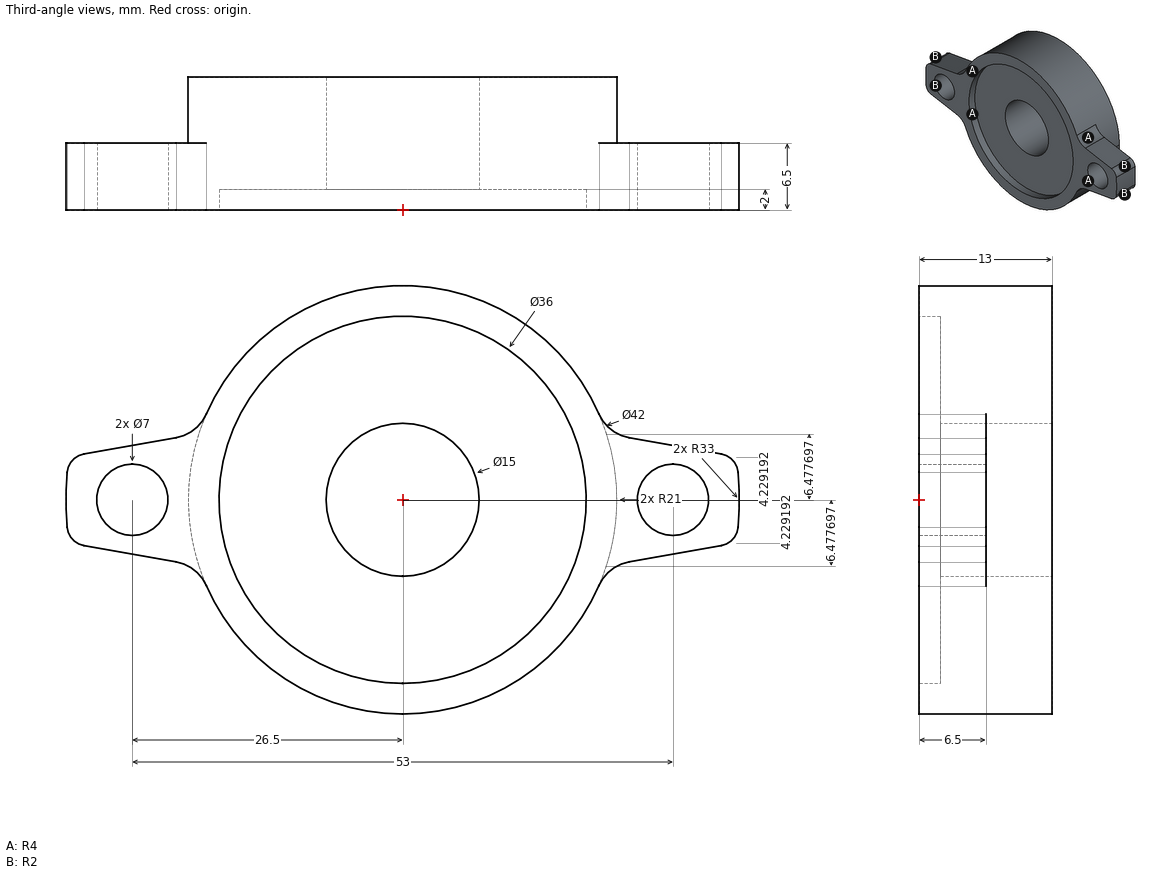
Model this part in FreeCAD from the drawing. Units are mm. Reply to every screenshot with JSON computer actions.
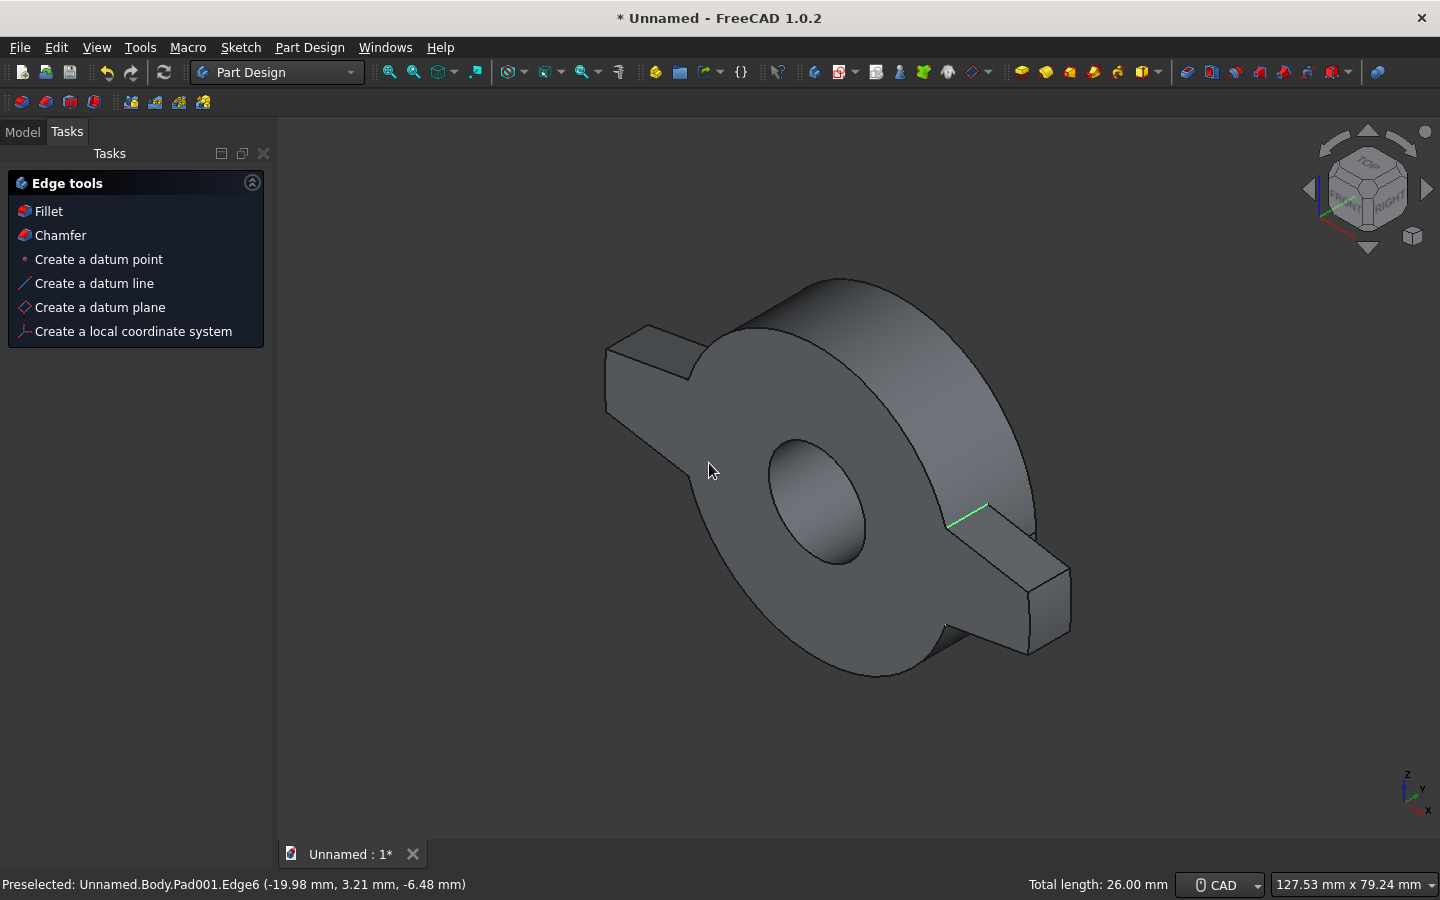
{"action": "left_click", "coordinate": [22, 102]}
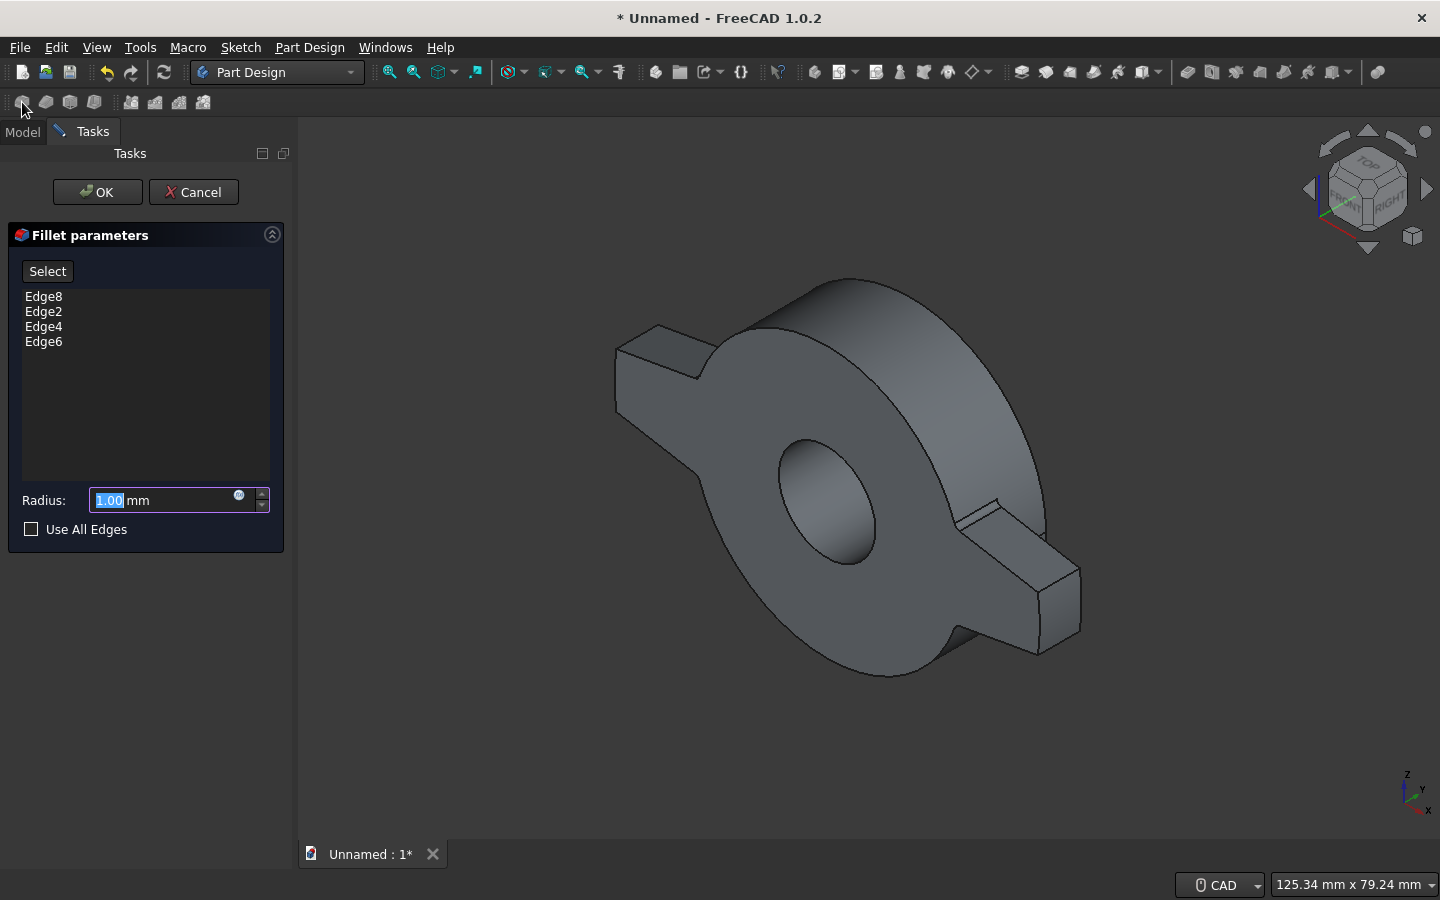
{"action": "type", "text": "4"}
{"action": "key", "text": "Tab"}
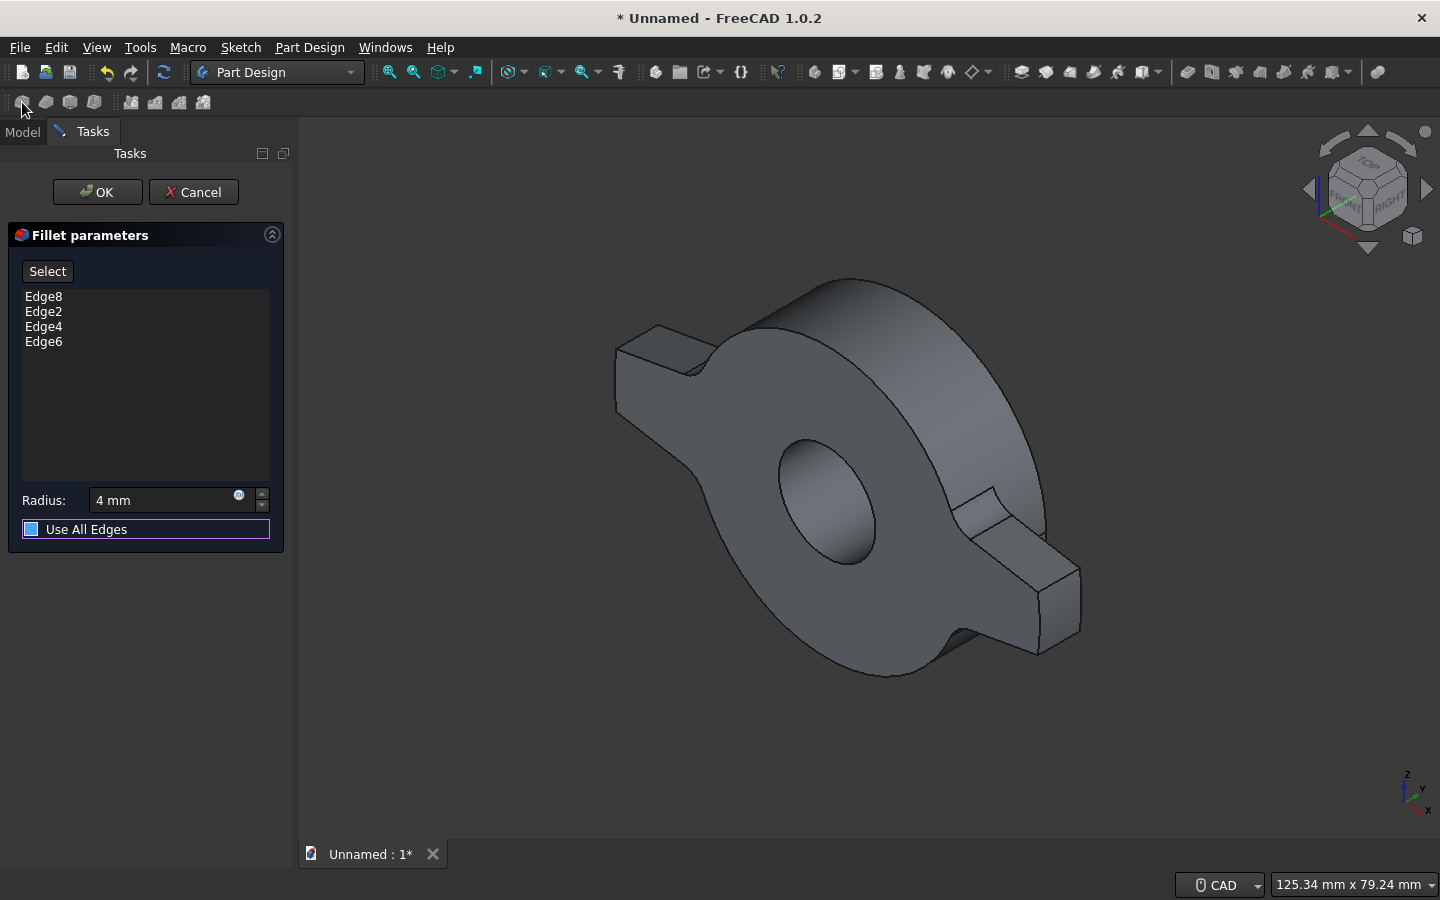
{"action": "left_click", "coordinate": [98, 192]}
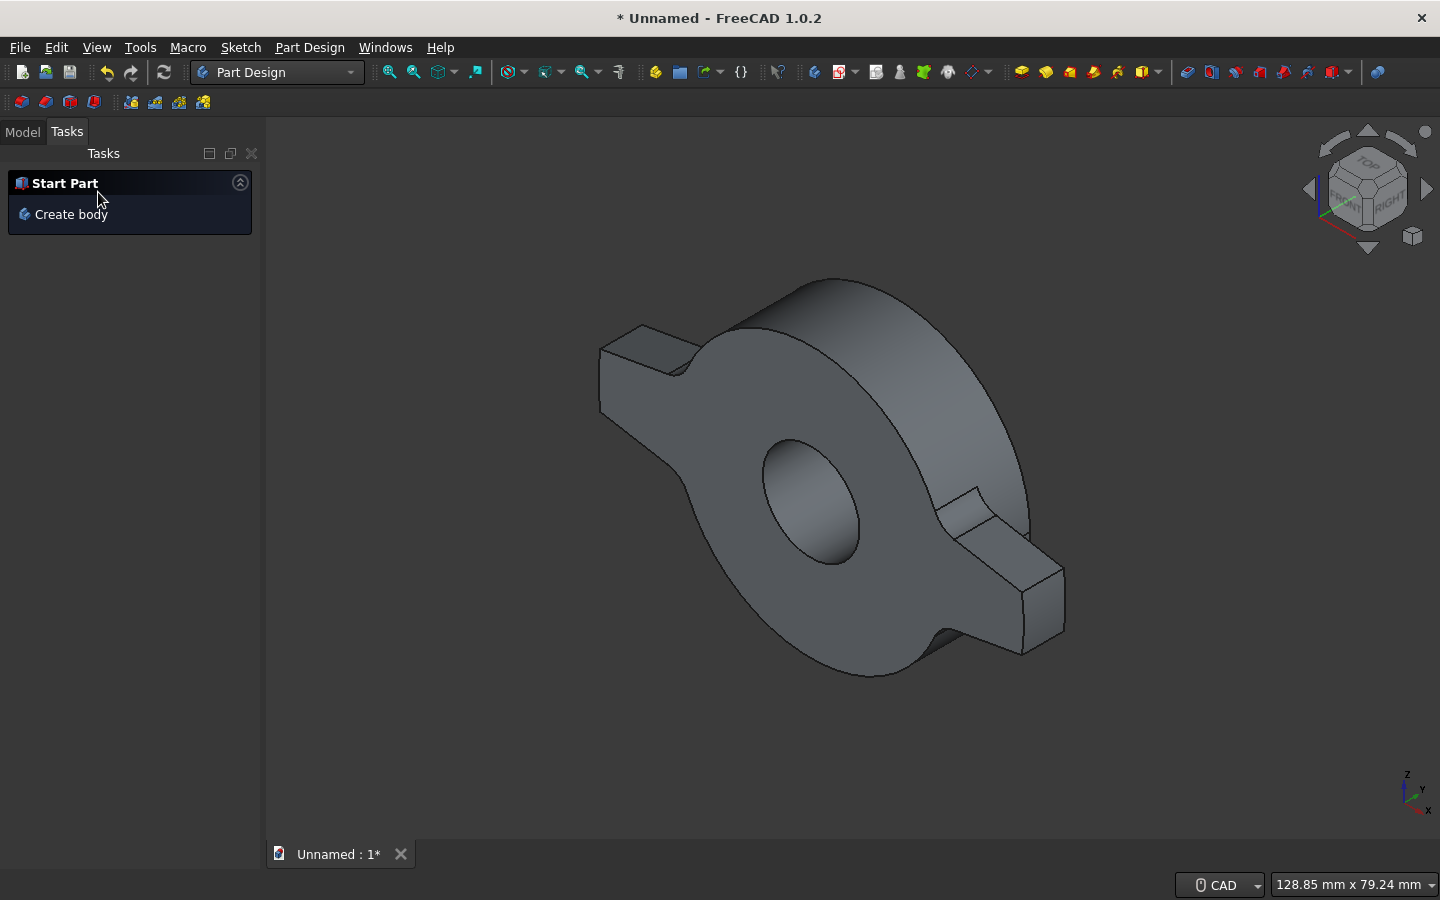
{"action": "left_click", "coordinate": [1043, 579]}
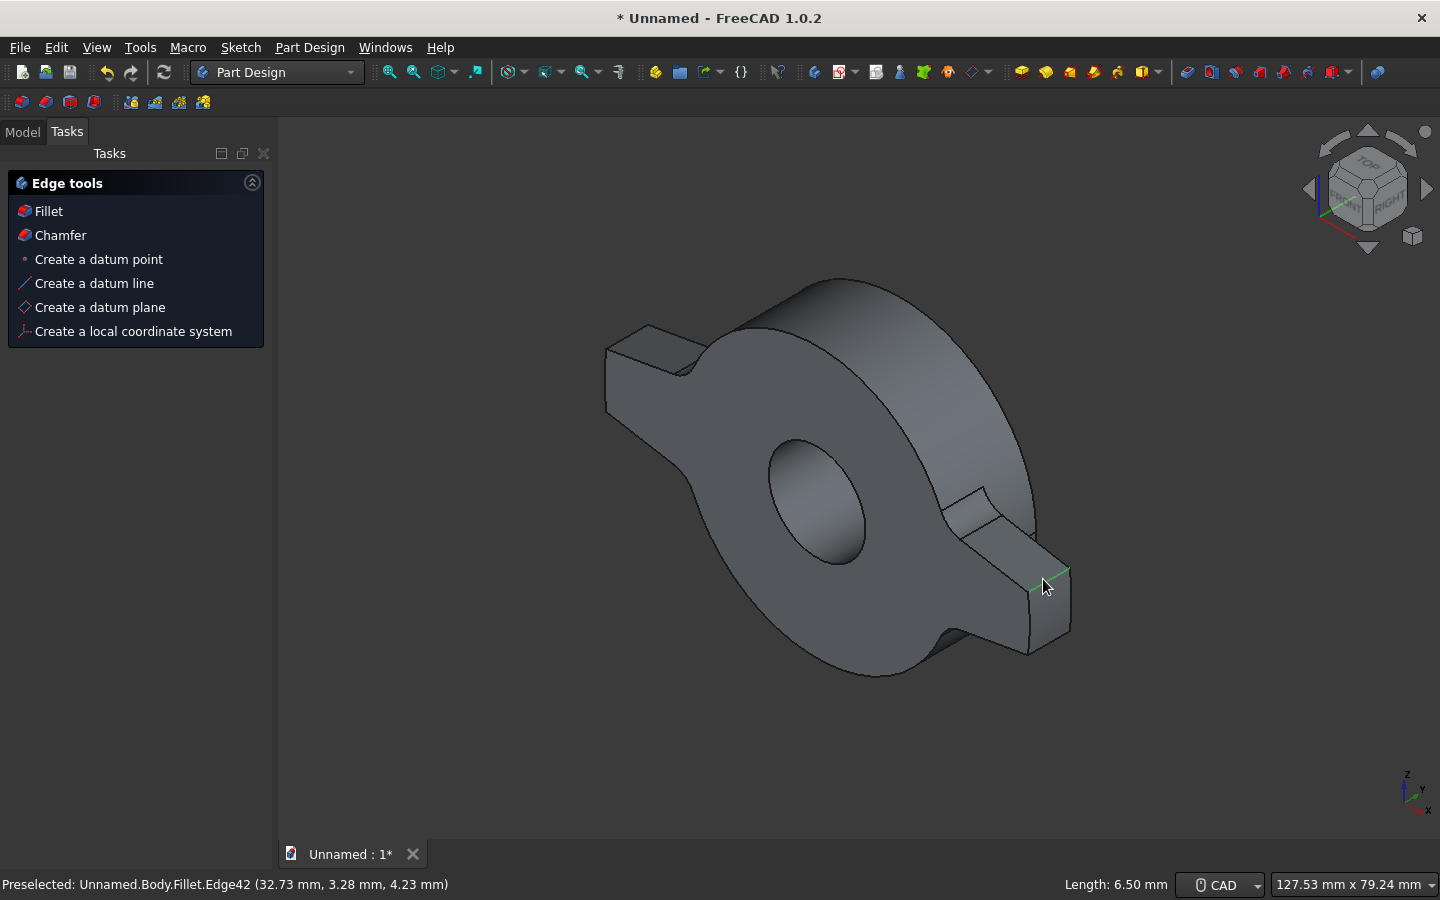
{"action": "key", "text": "2"}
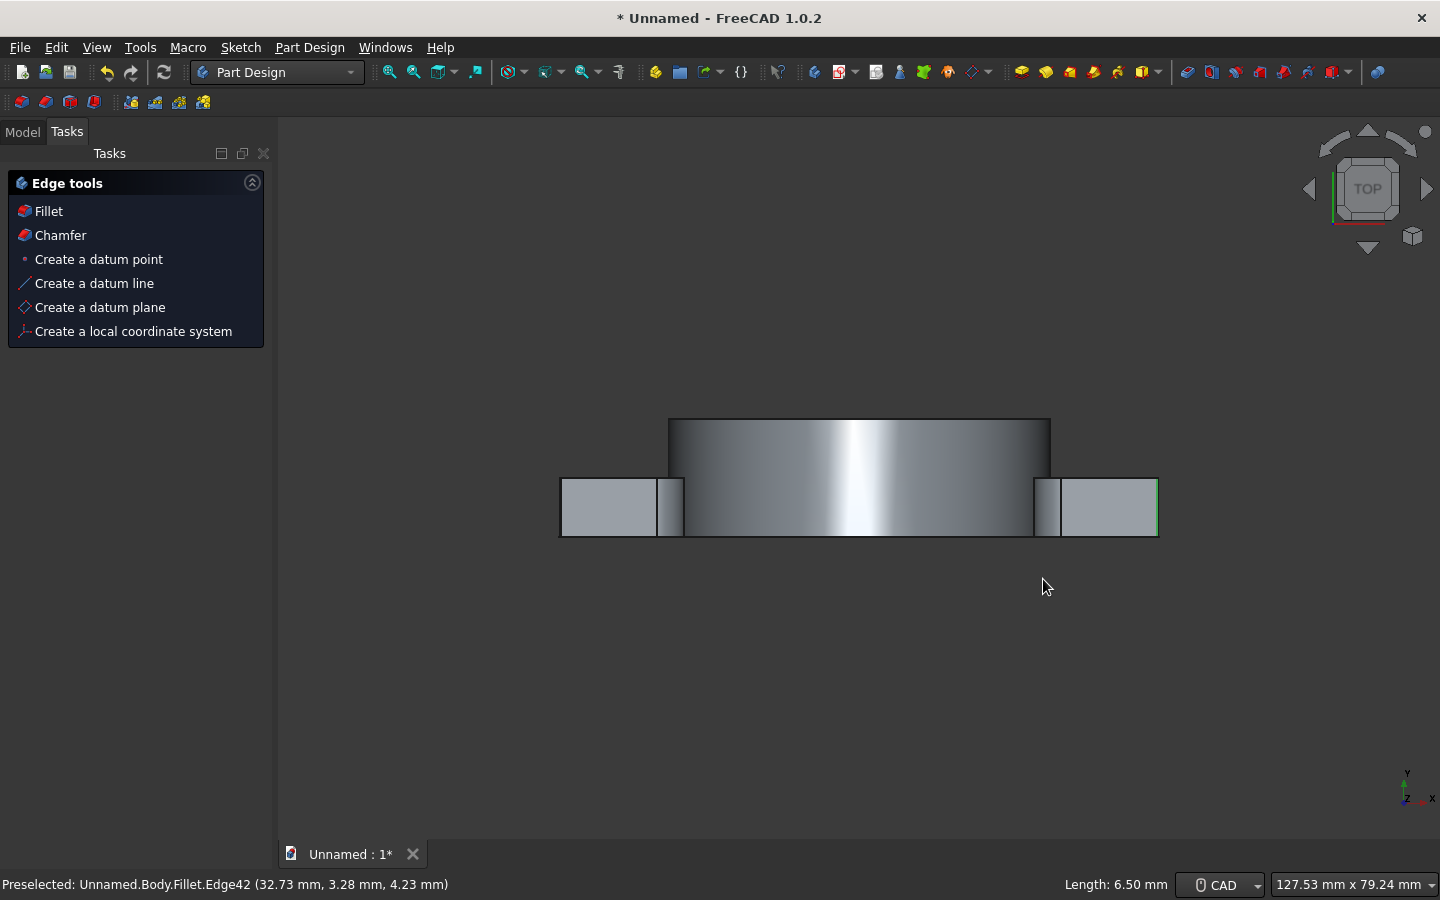
{"action": "key", "text": "0"}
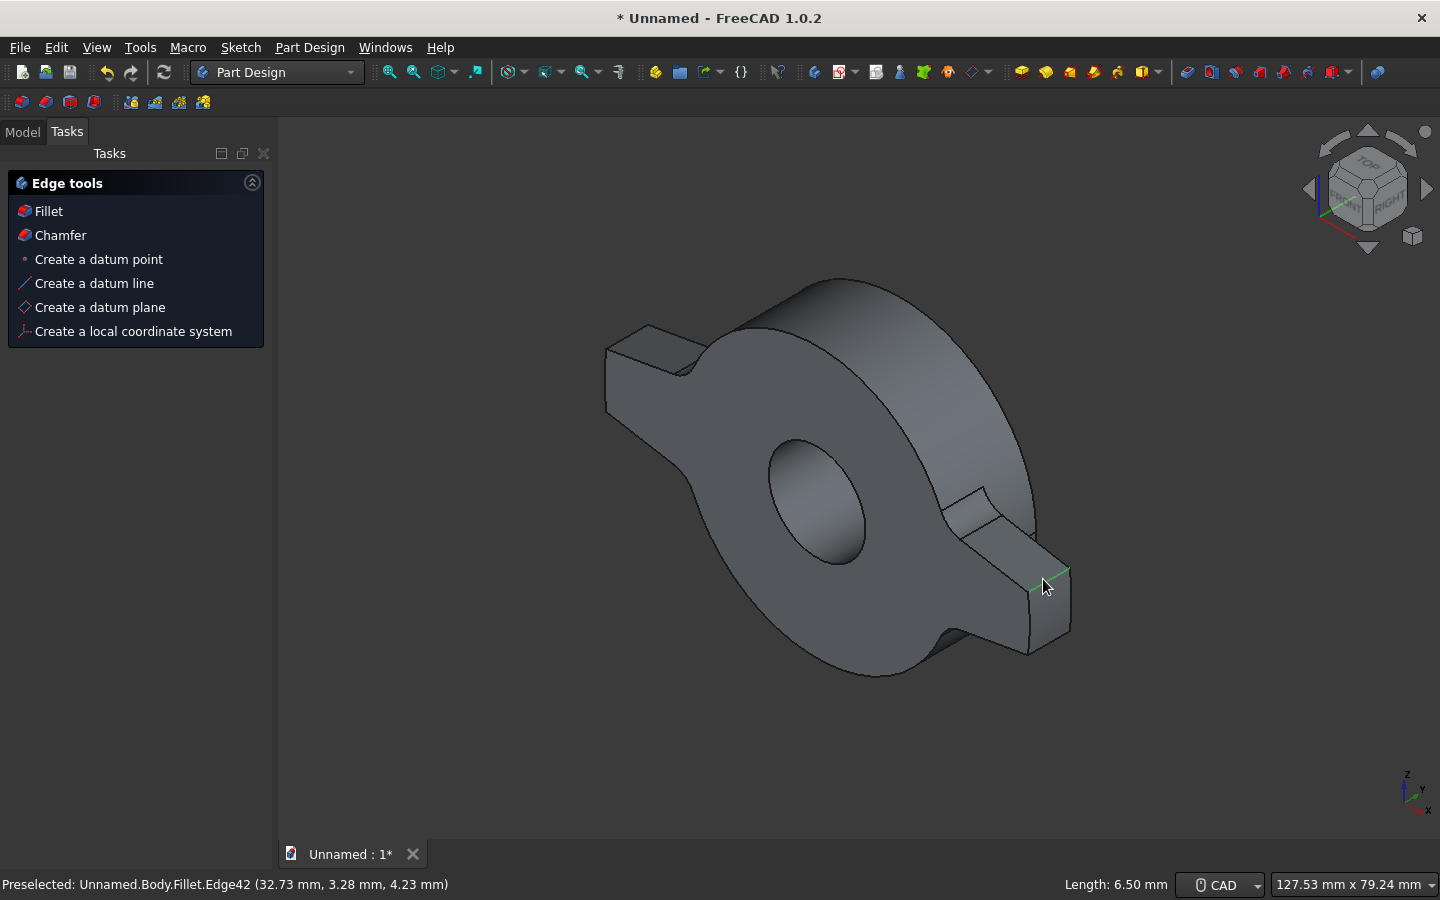
{"action": "key", "text": "1"}